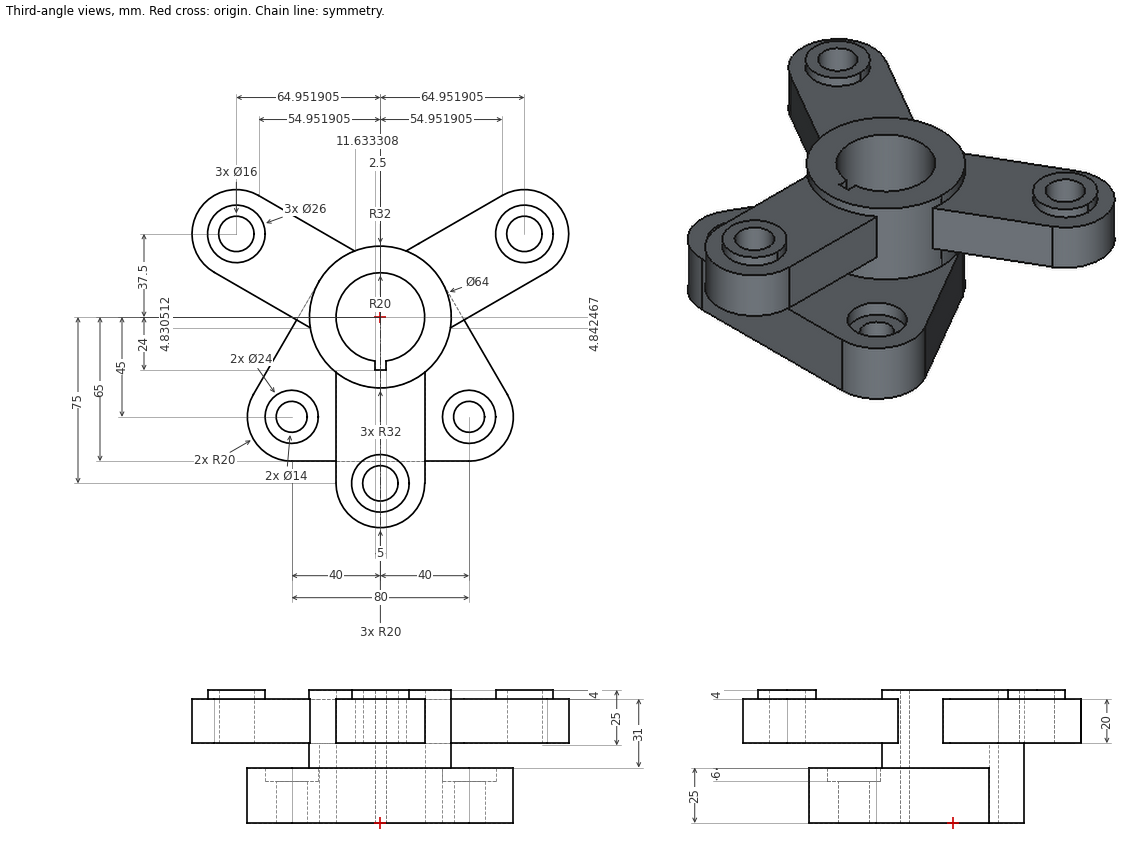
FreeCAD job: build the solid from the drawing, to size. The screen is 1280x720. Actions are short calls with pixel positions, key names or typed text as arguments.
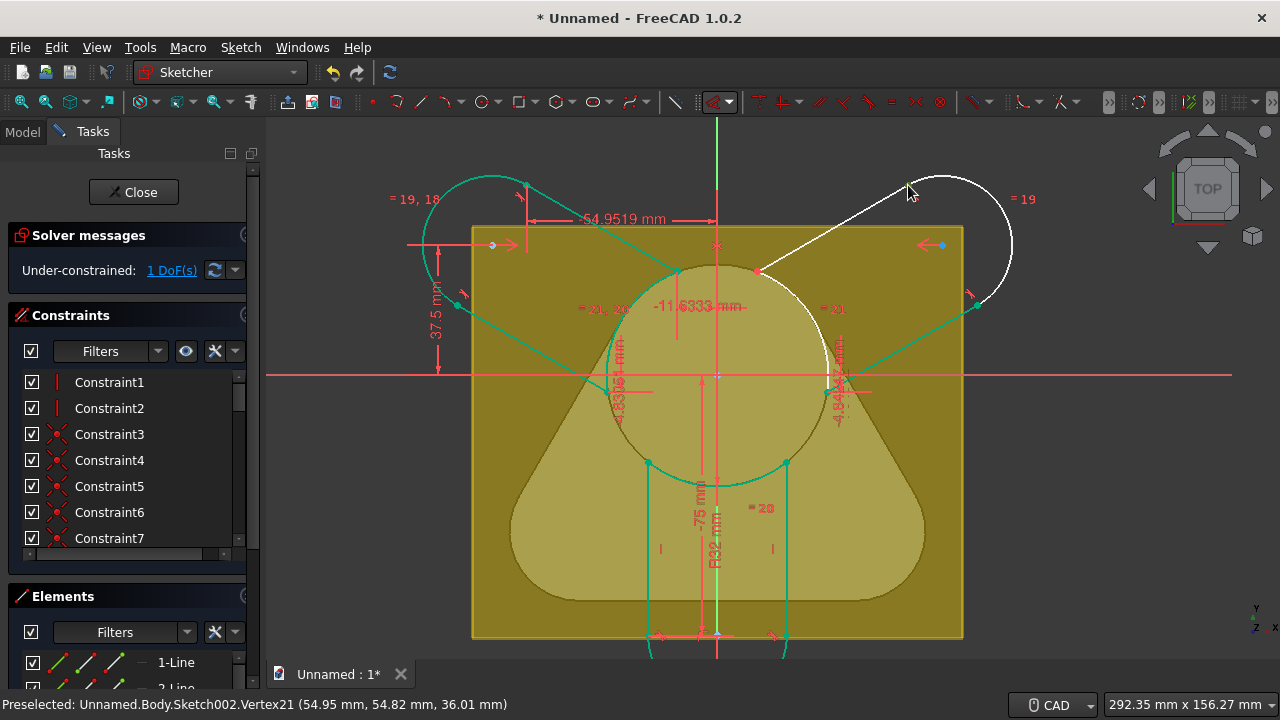
click(732, 102)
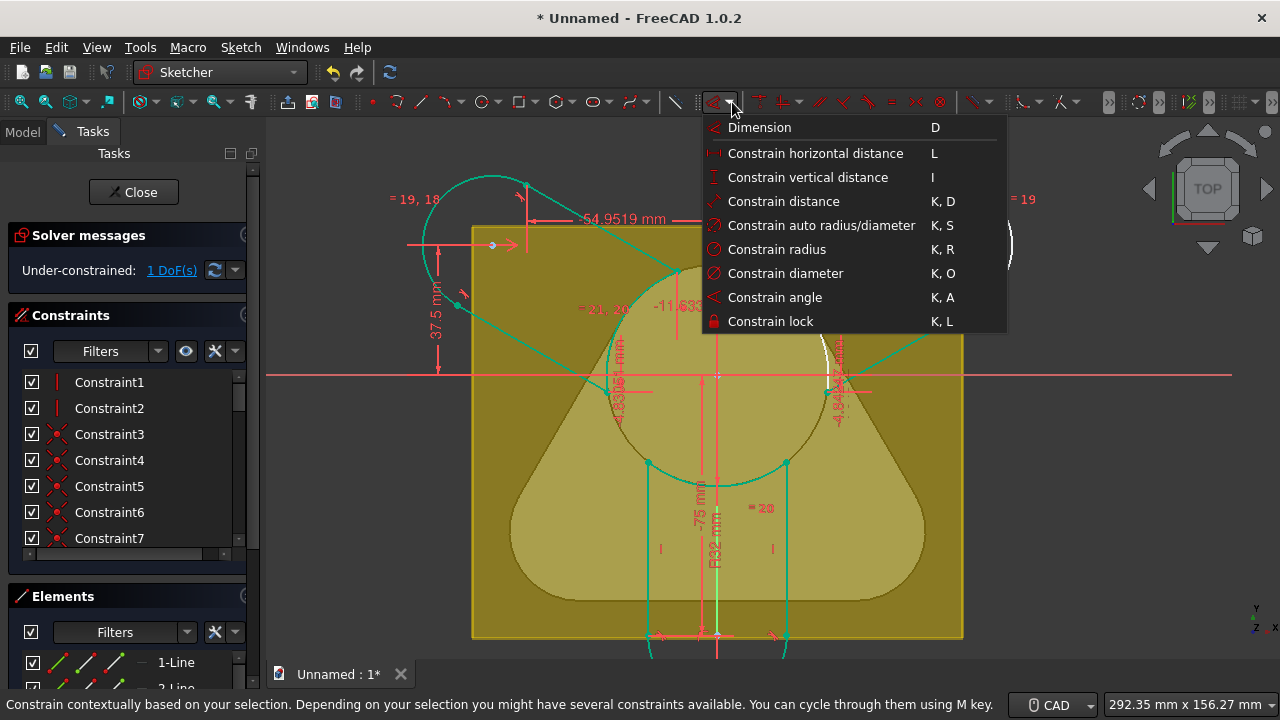
click(855, 153)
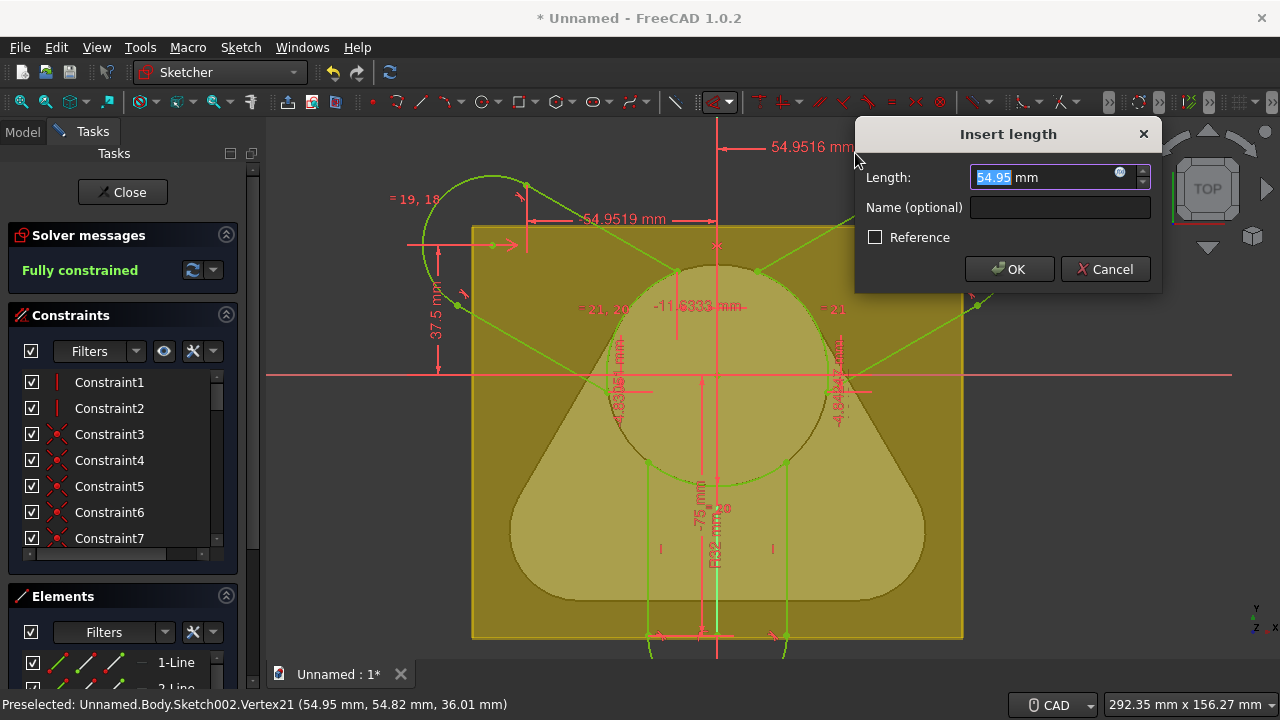
text(54.951905)
key(Return)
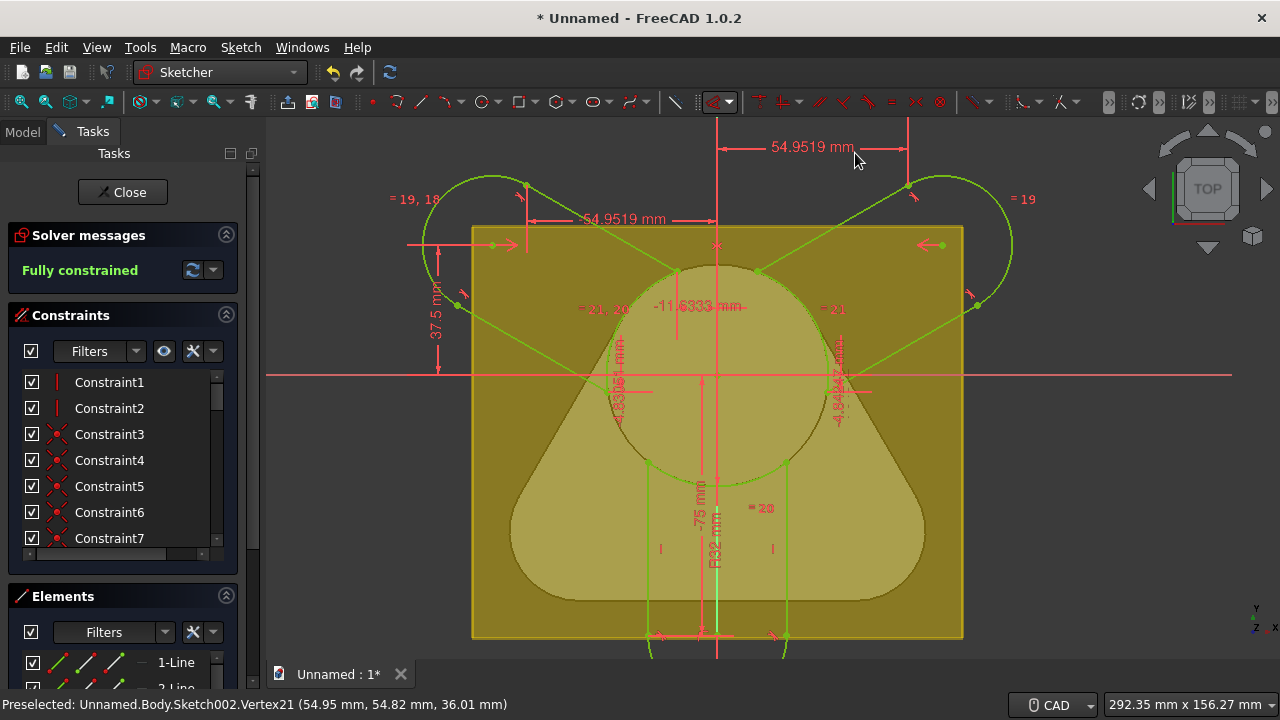
click(123, 192)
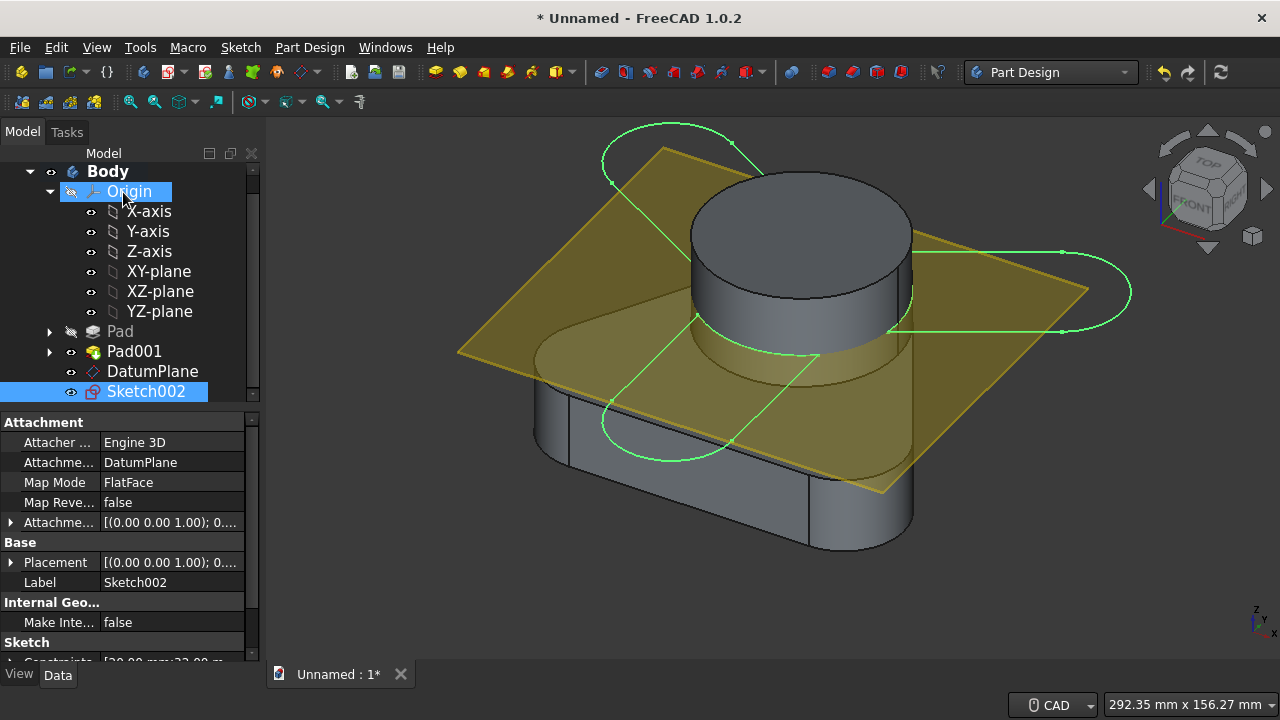
click(436, 72)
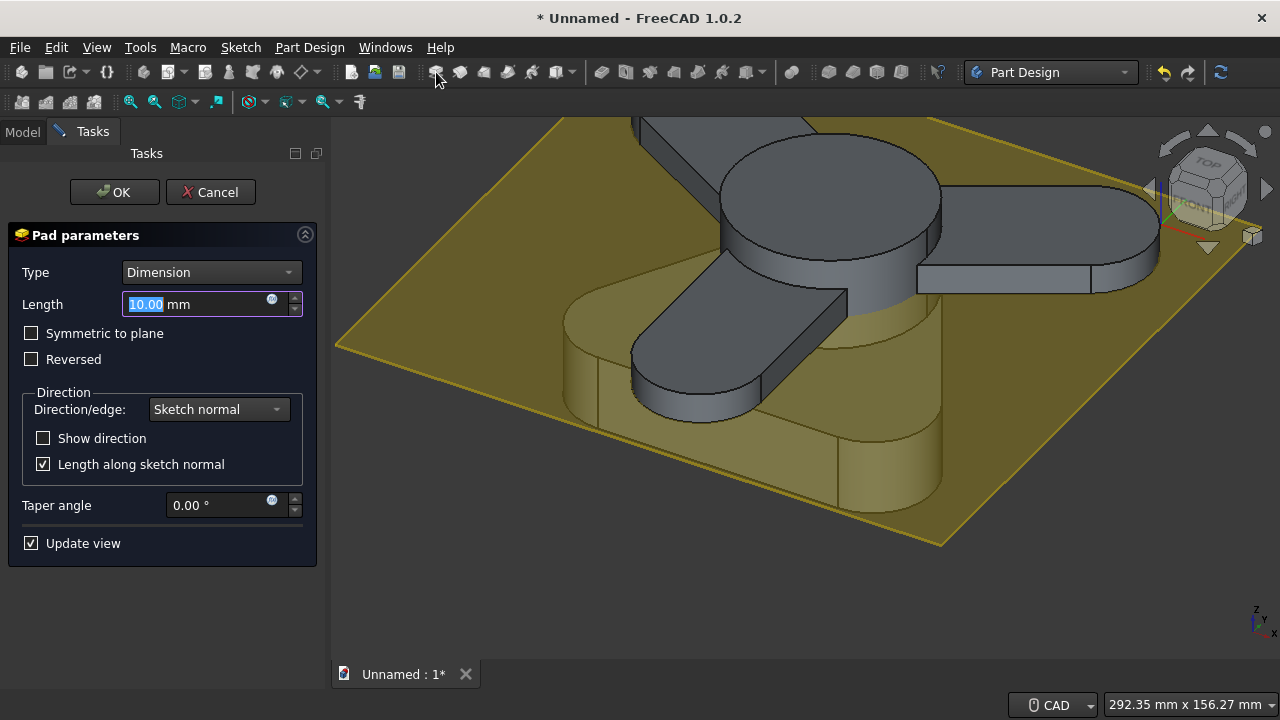
text(20)
key(Tab)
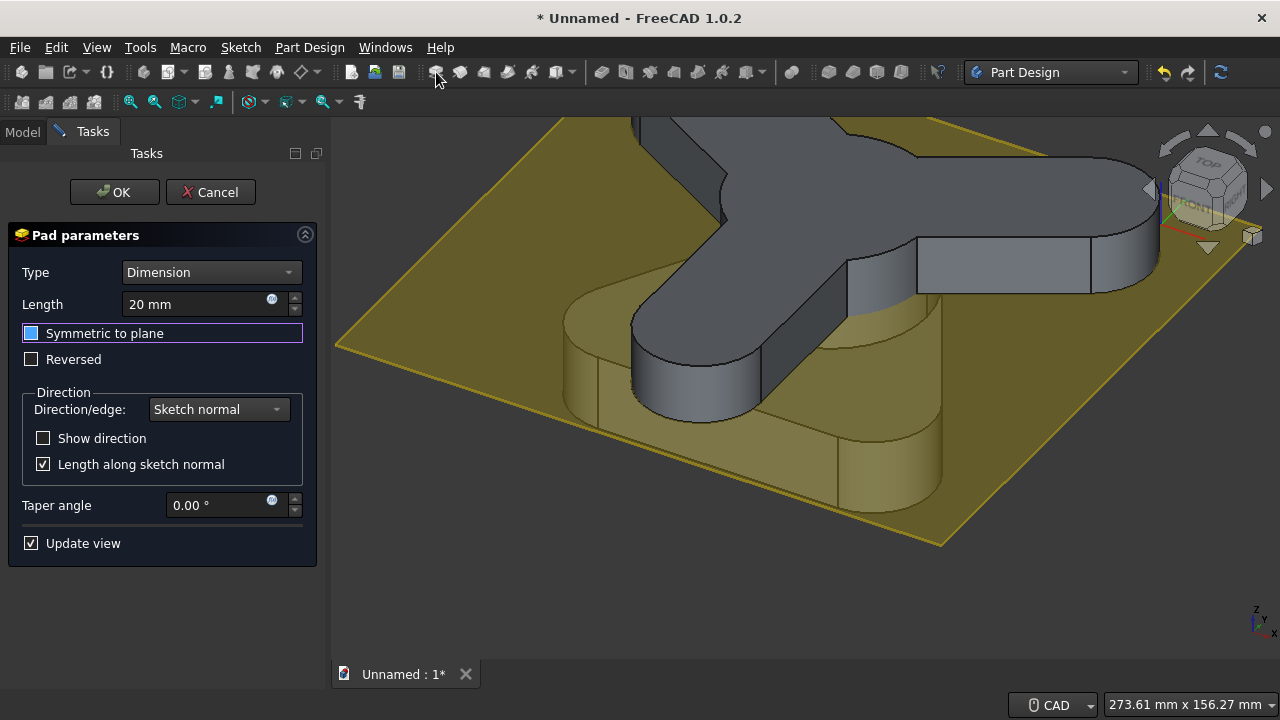
click(115, 192)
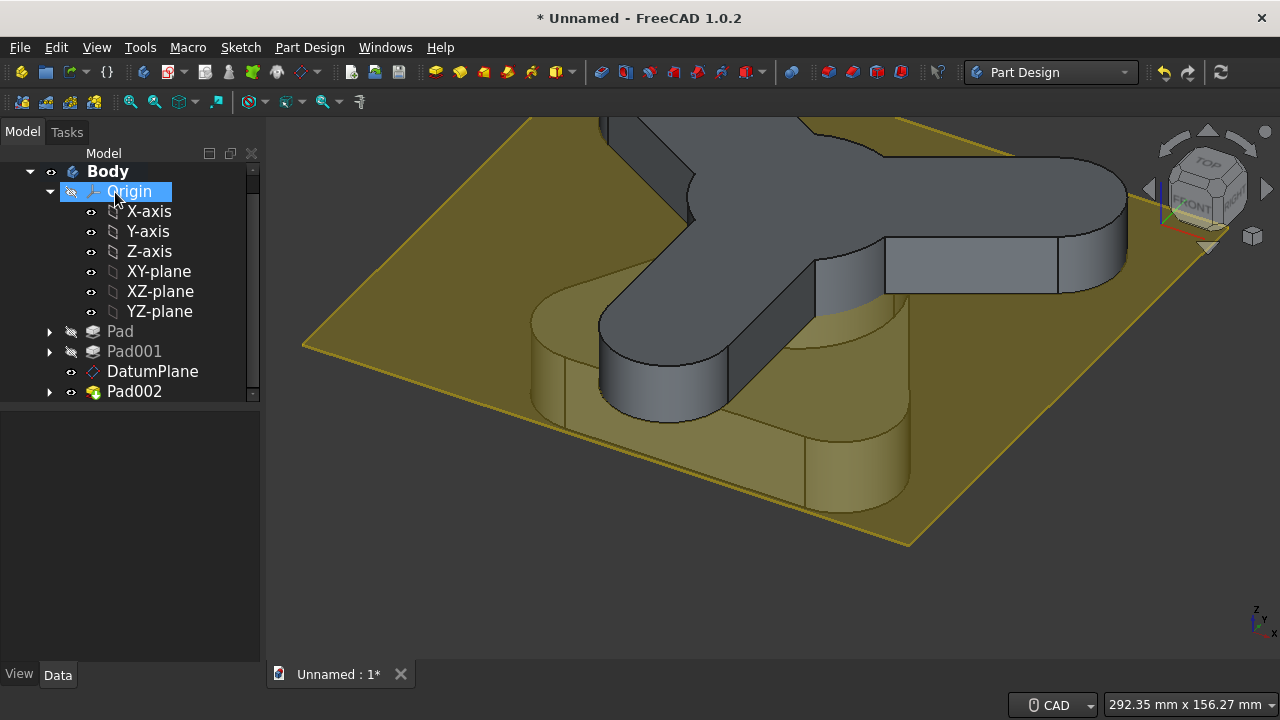
click(116, 372)
key(space)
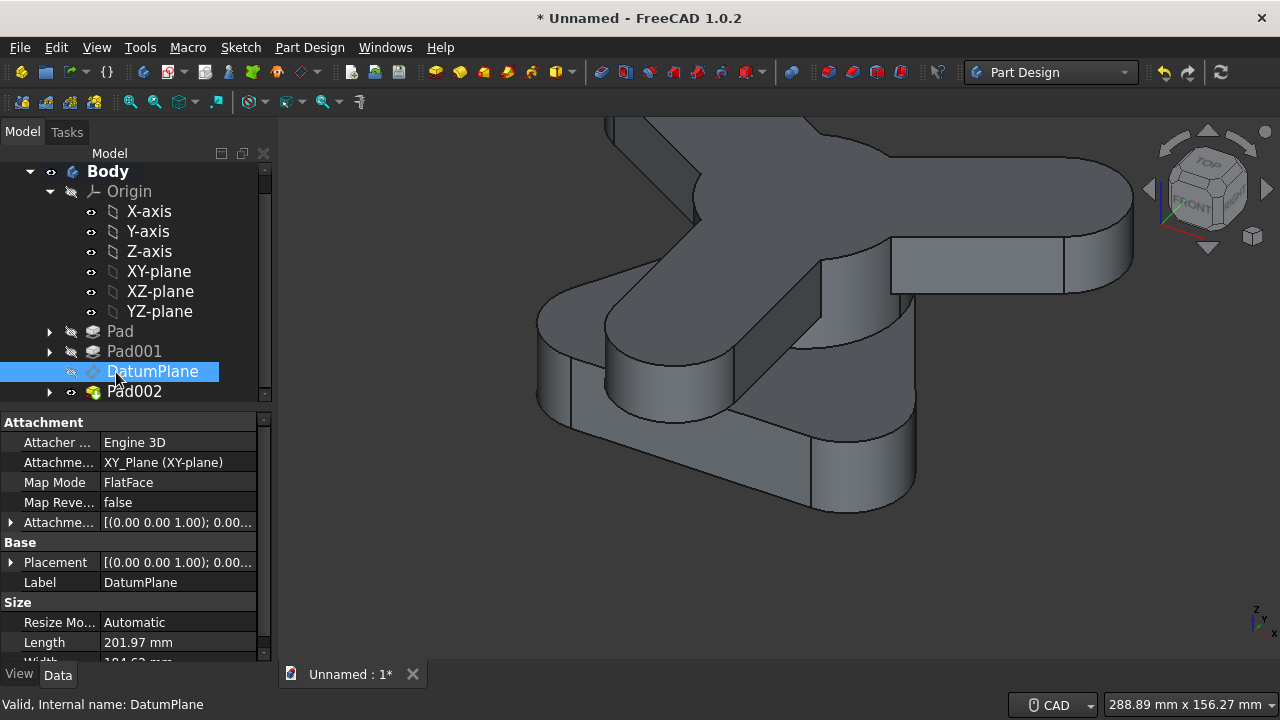
key(v)
key(f)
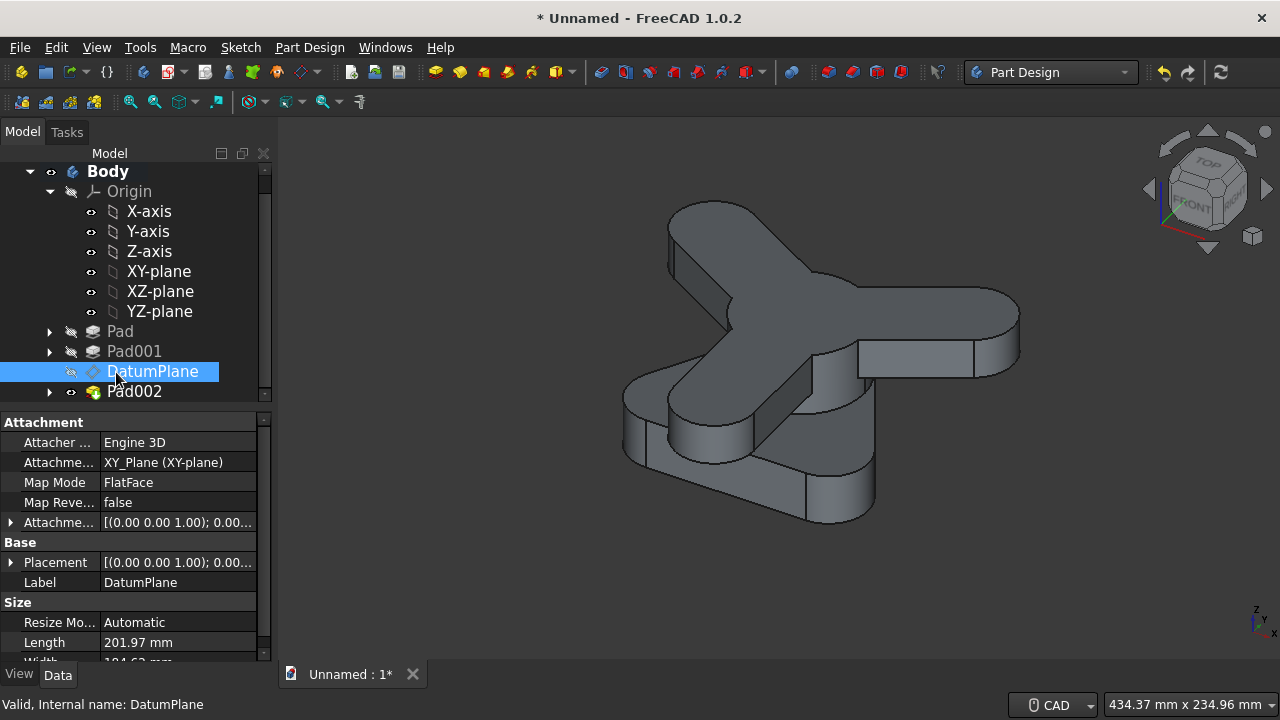
click(804, 309)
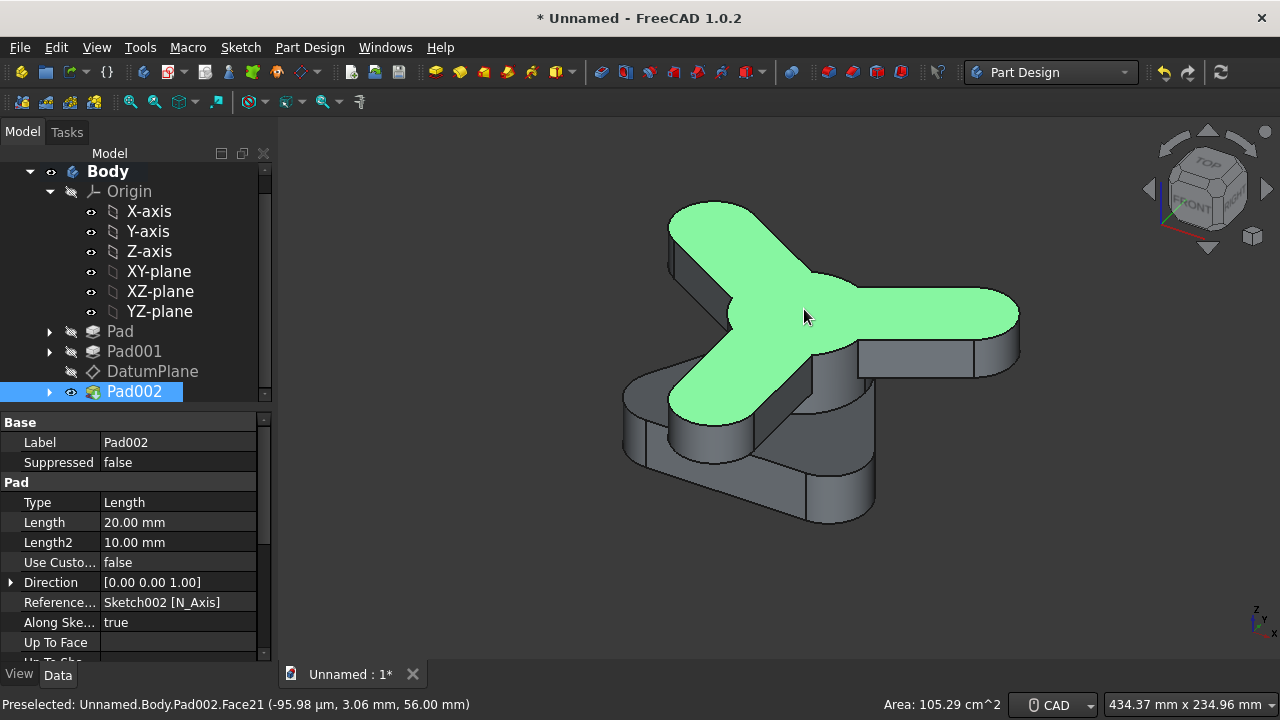
click(168, 72)